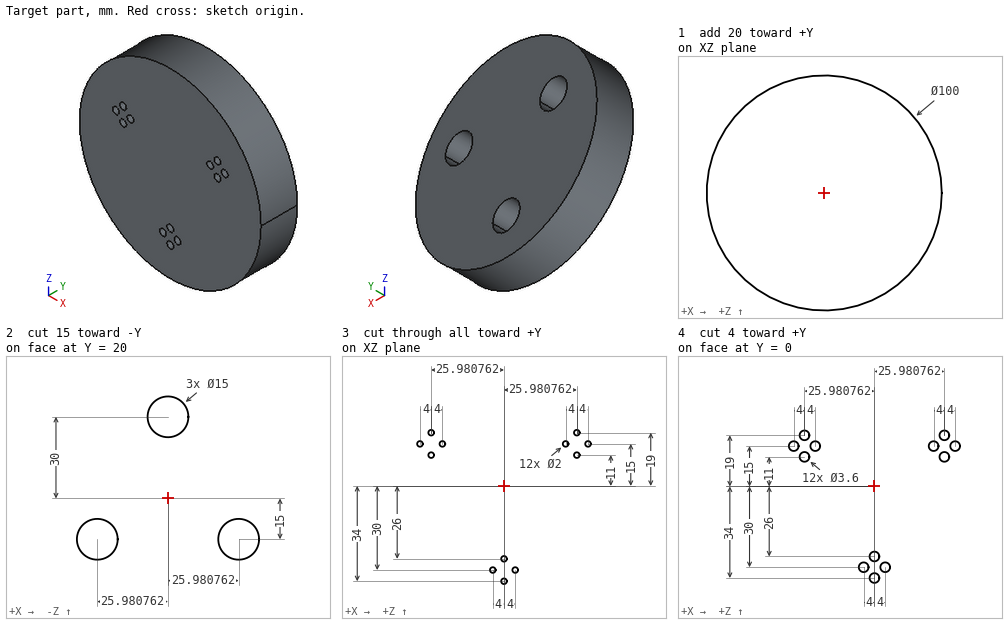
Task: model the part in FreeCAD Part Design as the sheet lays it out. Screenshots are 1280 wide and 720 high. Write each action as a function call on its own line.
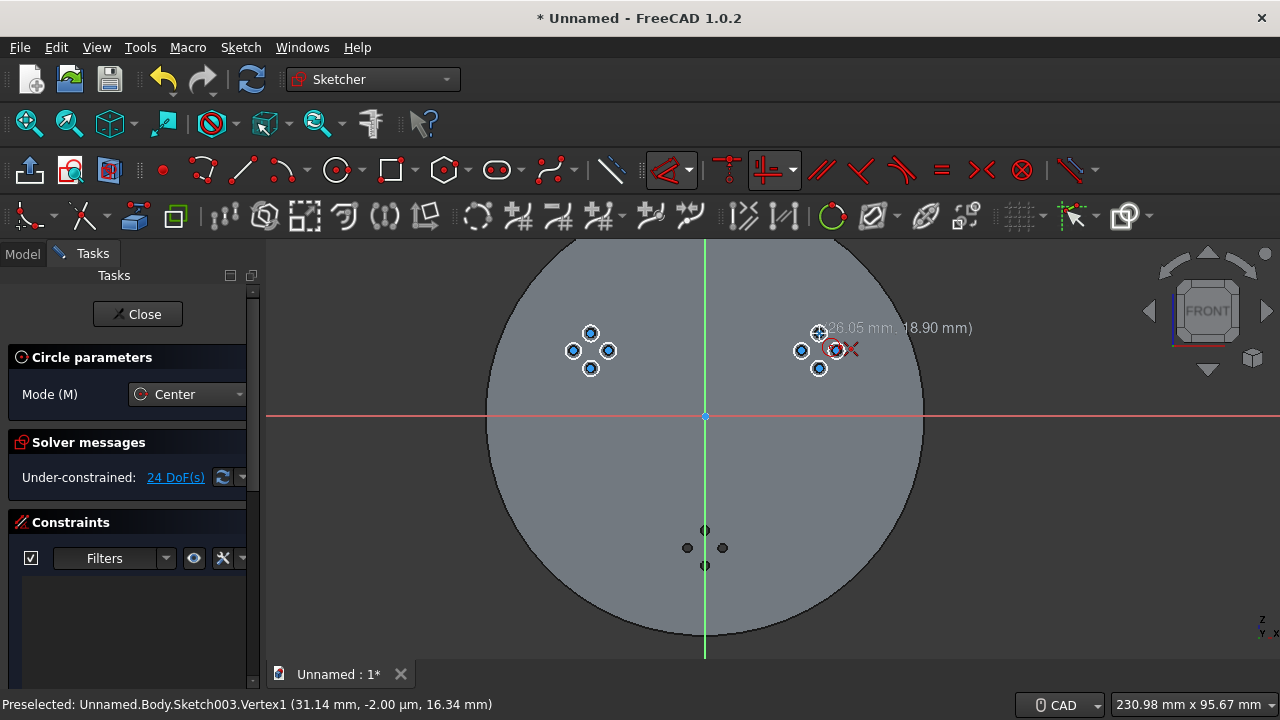
scroll(705, 531, up, 6)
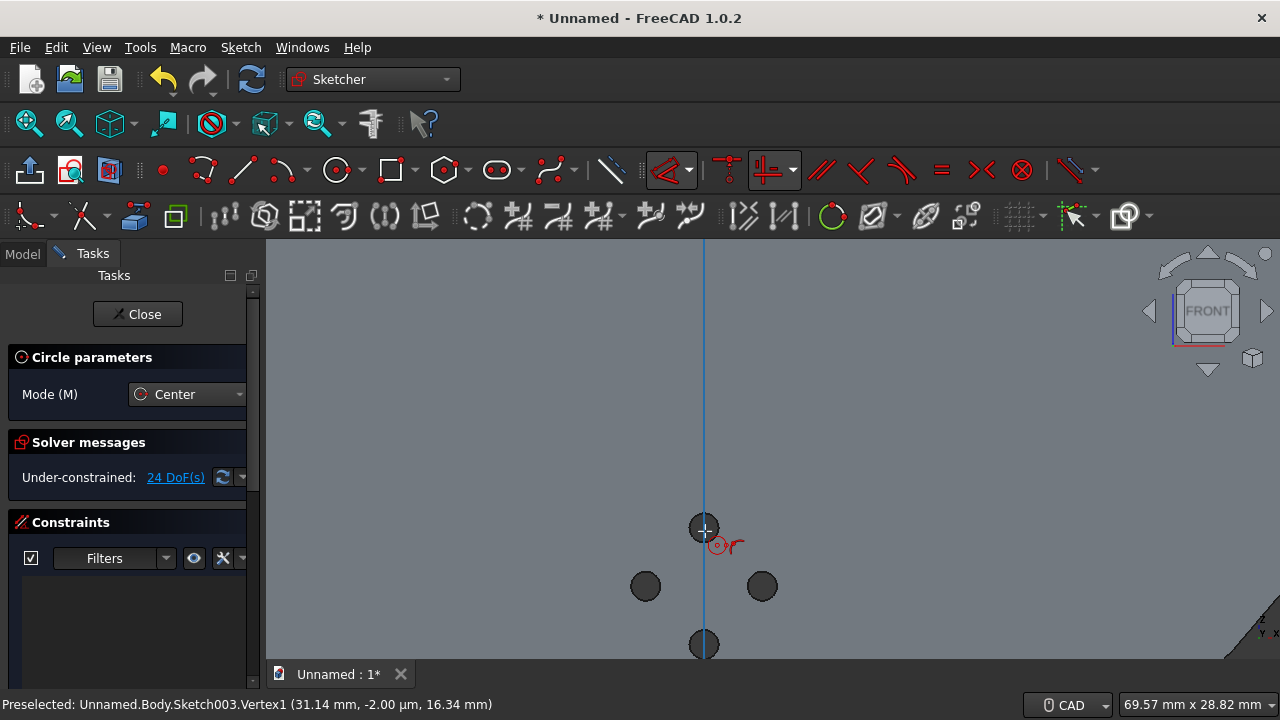
click(704, 528)
click(723, 509)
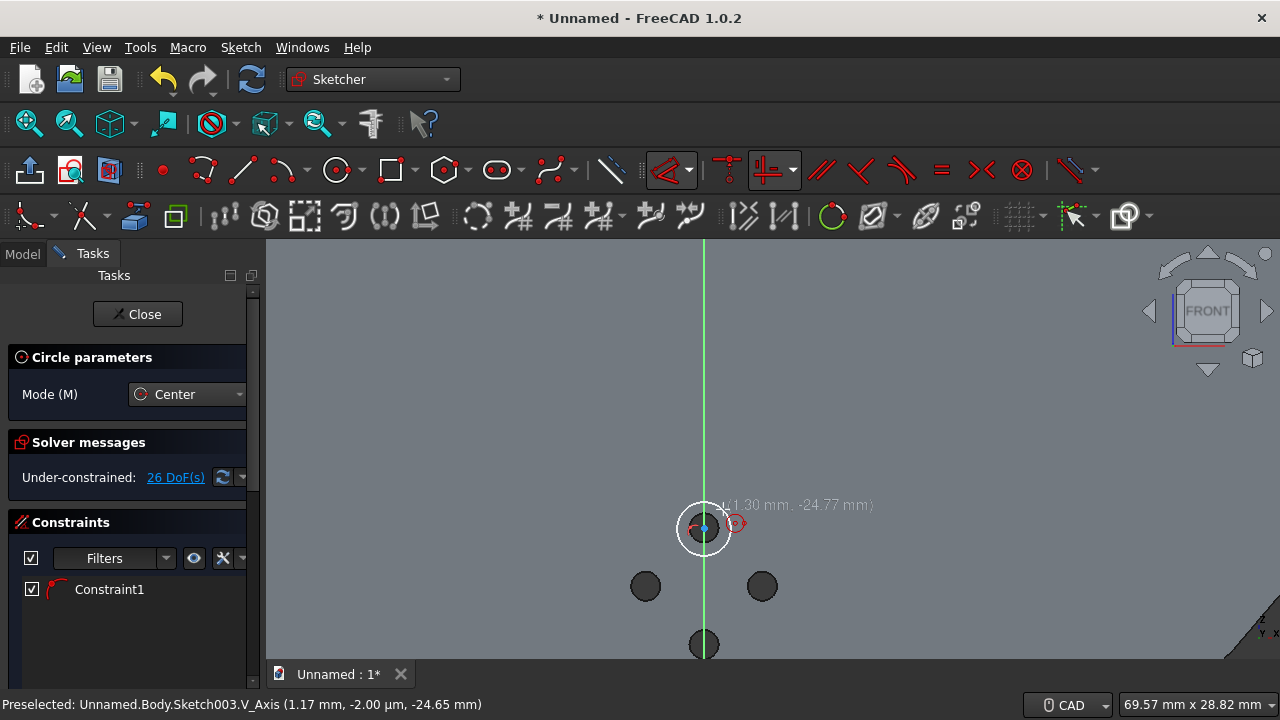
click(646, 586)
click(664, 568)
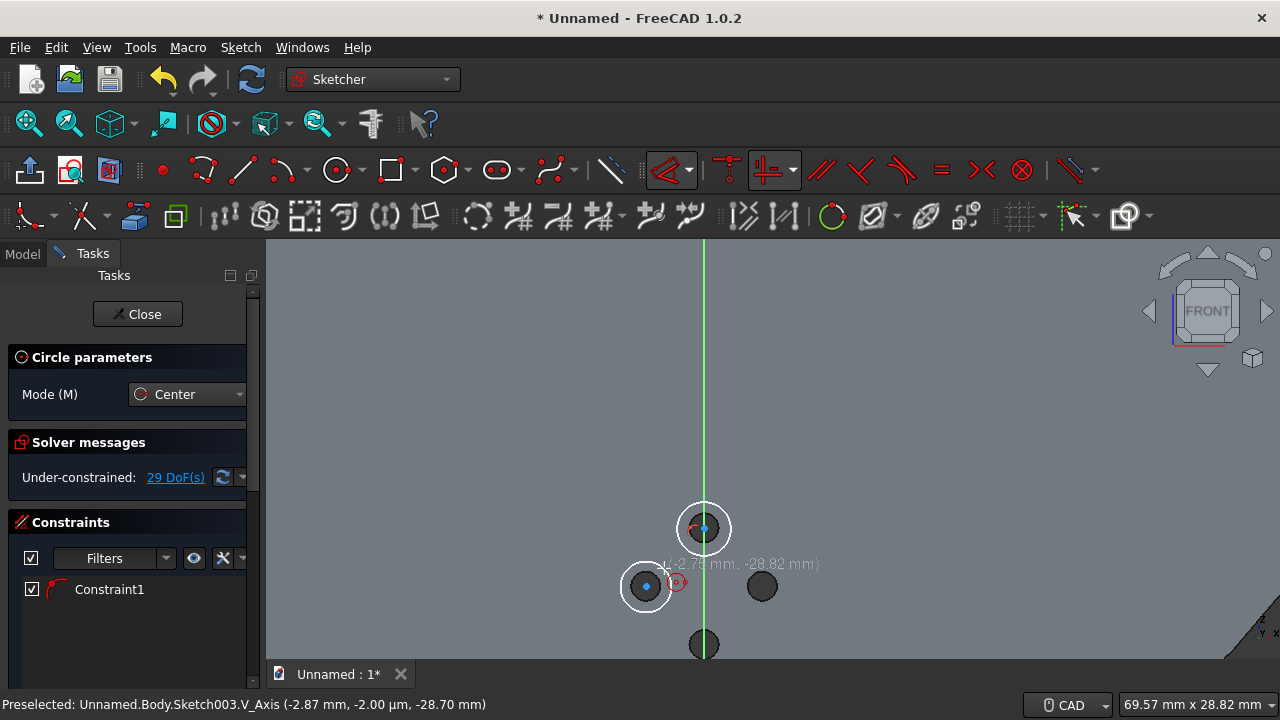
scroll(705, 531, down, 6)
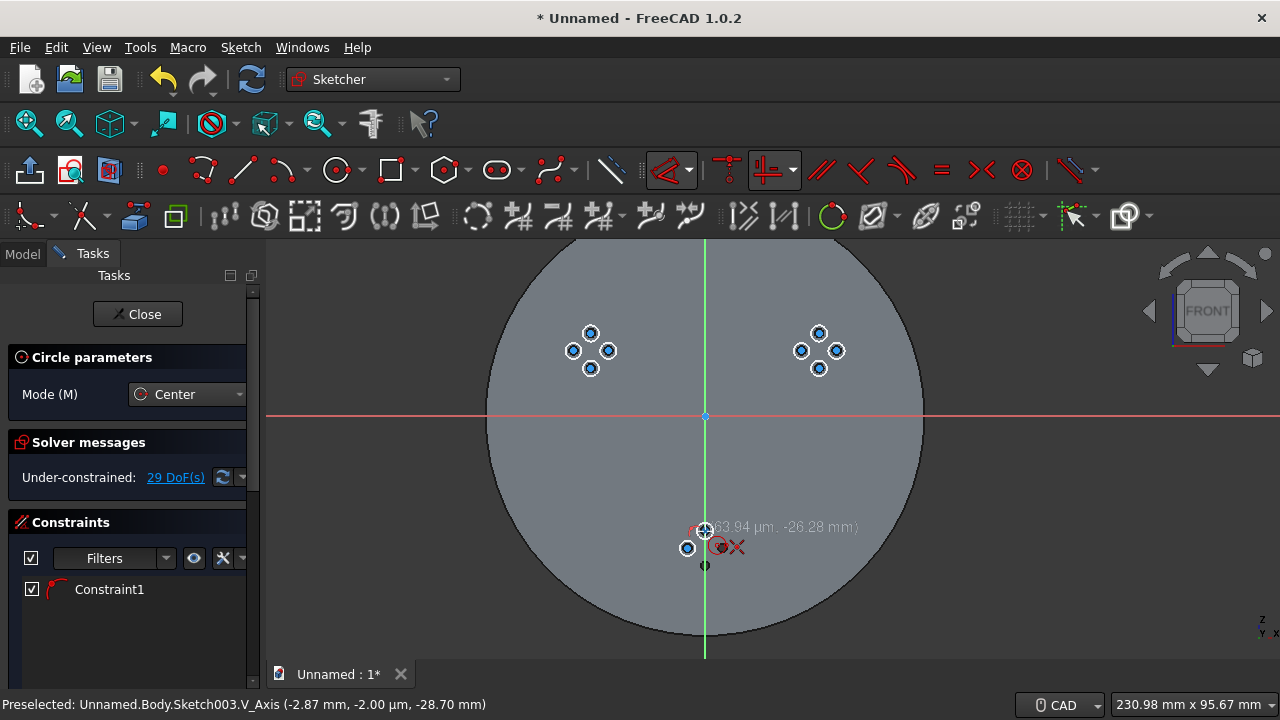
scroll(705, 566, up, 6)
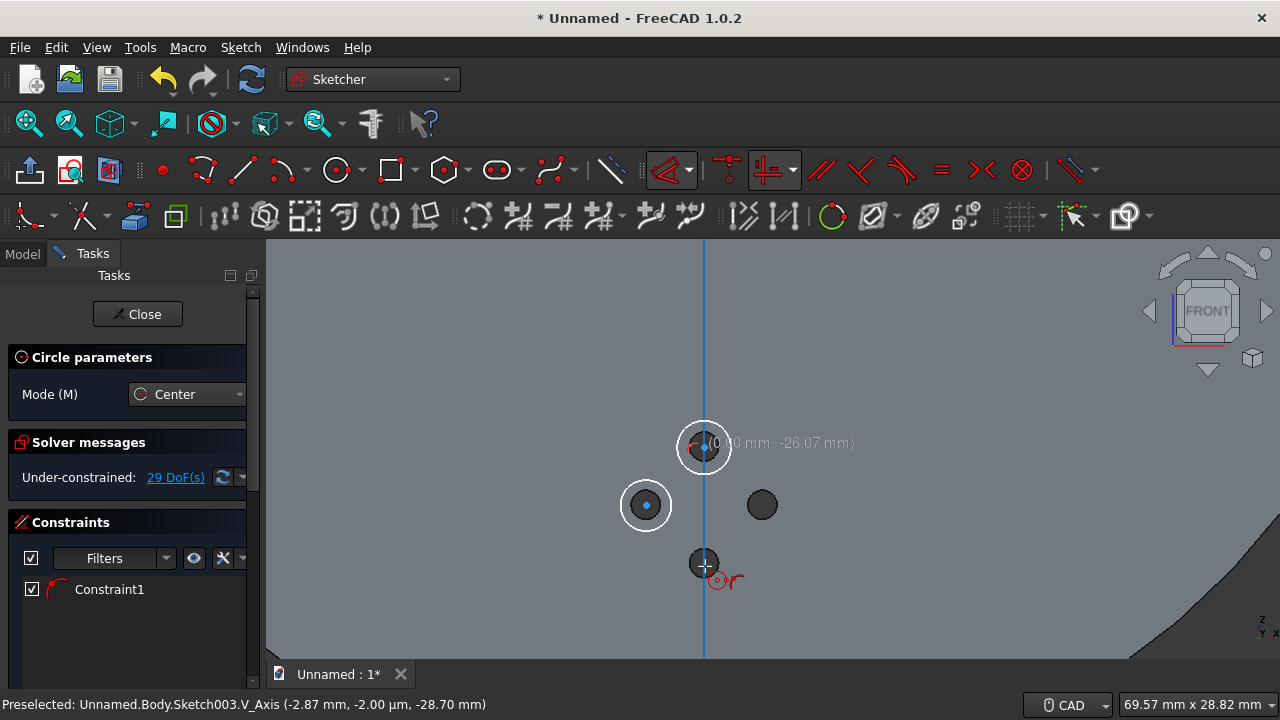
click(704, 563)
click(723, 545)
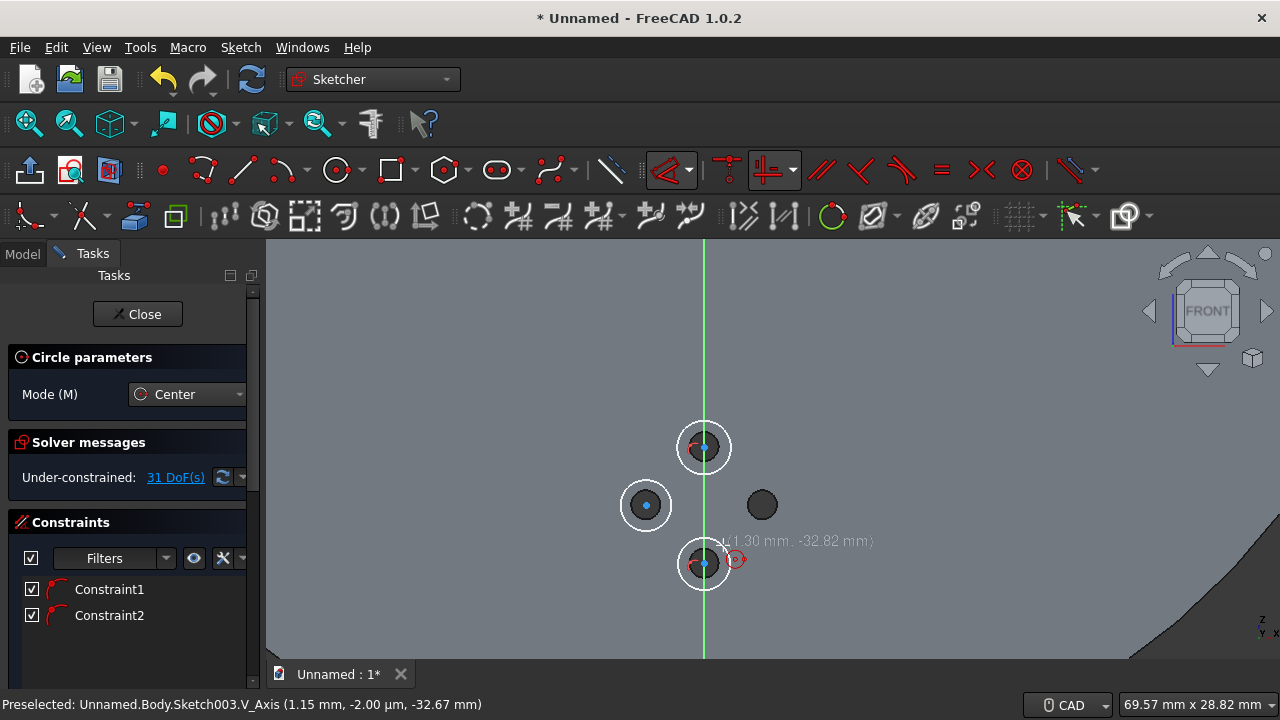
click(762, 505)
click(781, 486)
key(Escape)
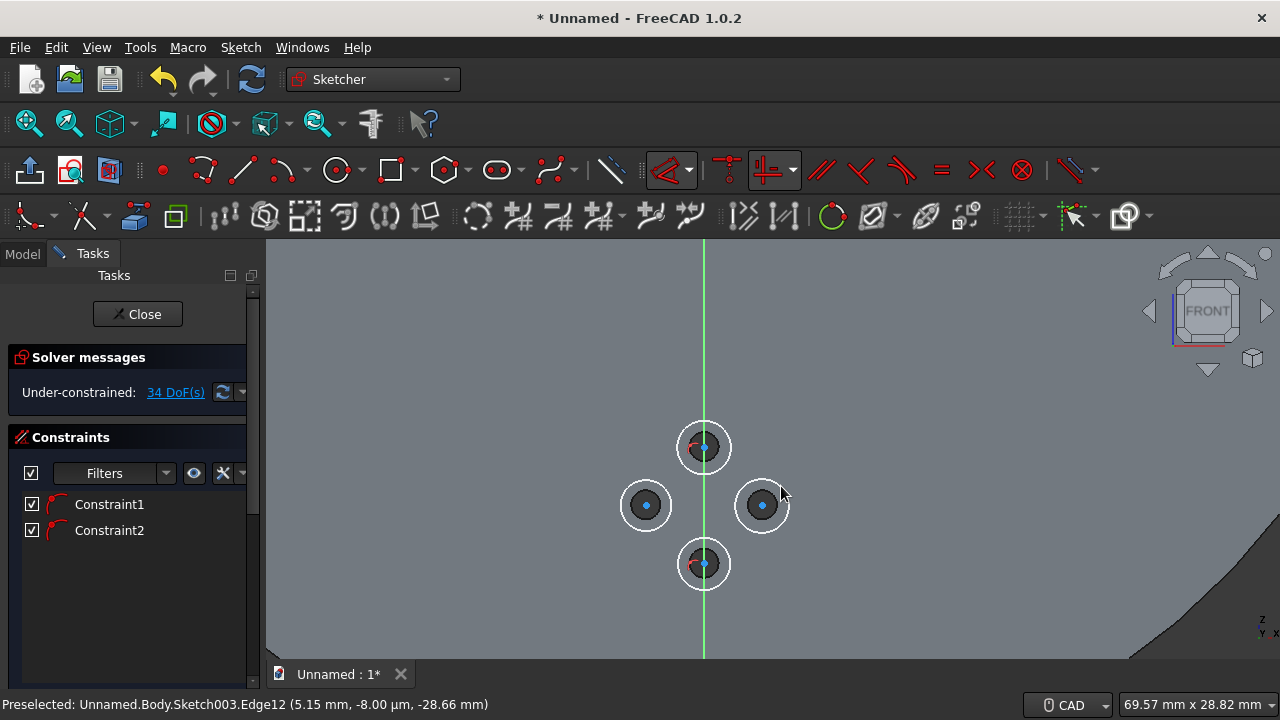
scroll(705, 566, down, 6)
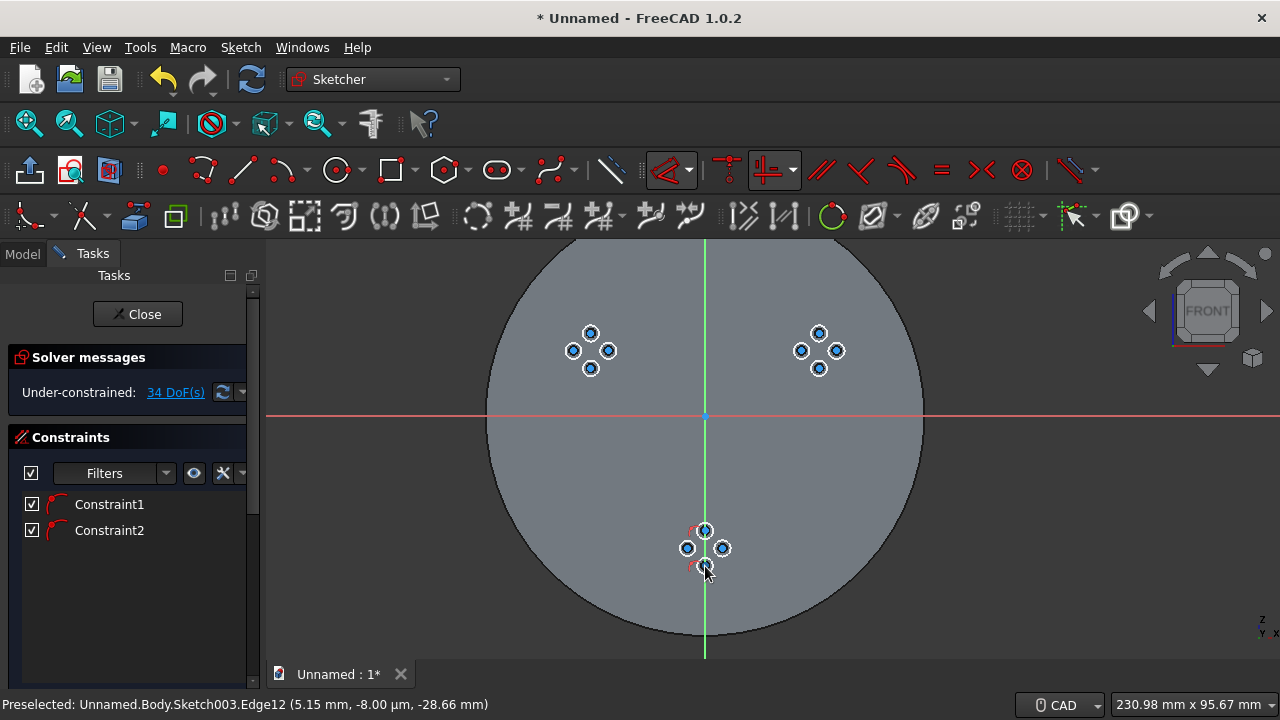
scroll(597, 328, up, 3)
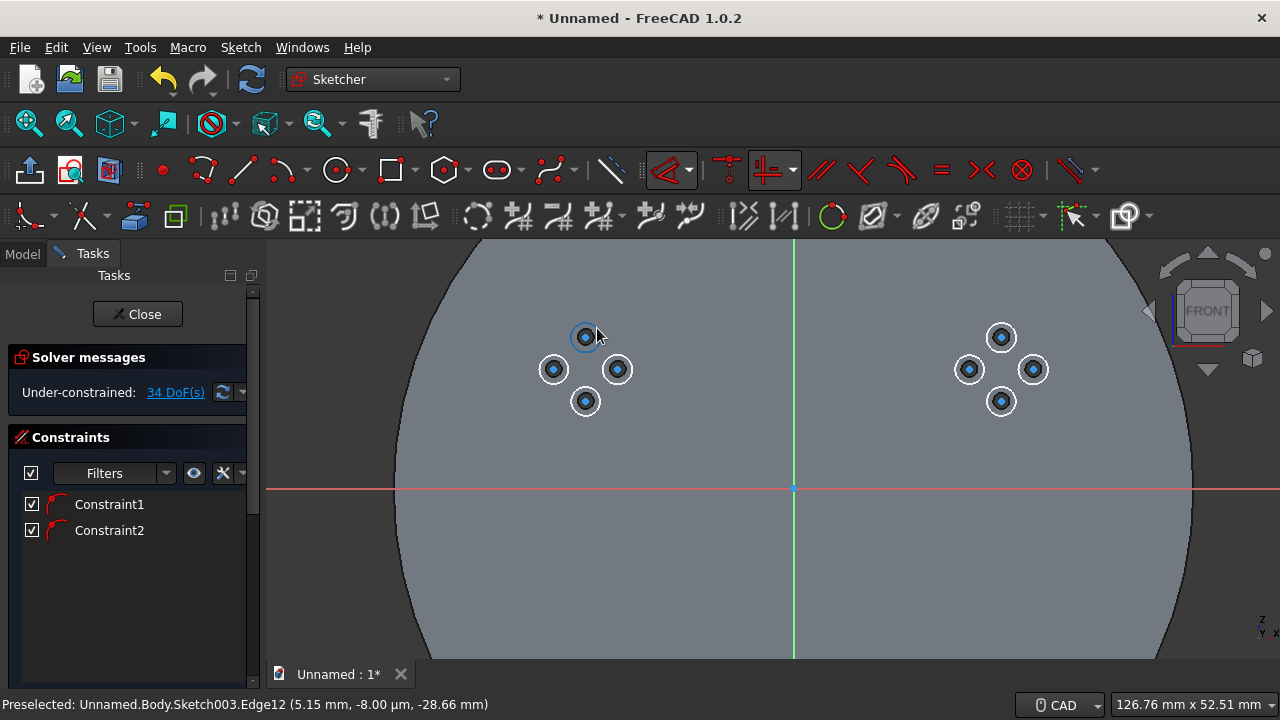
click(596, 327)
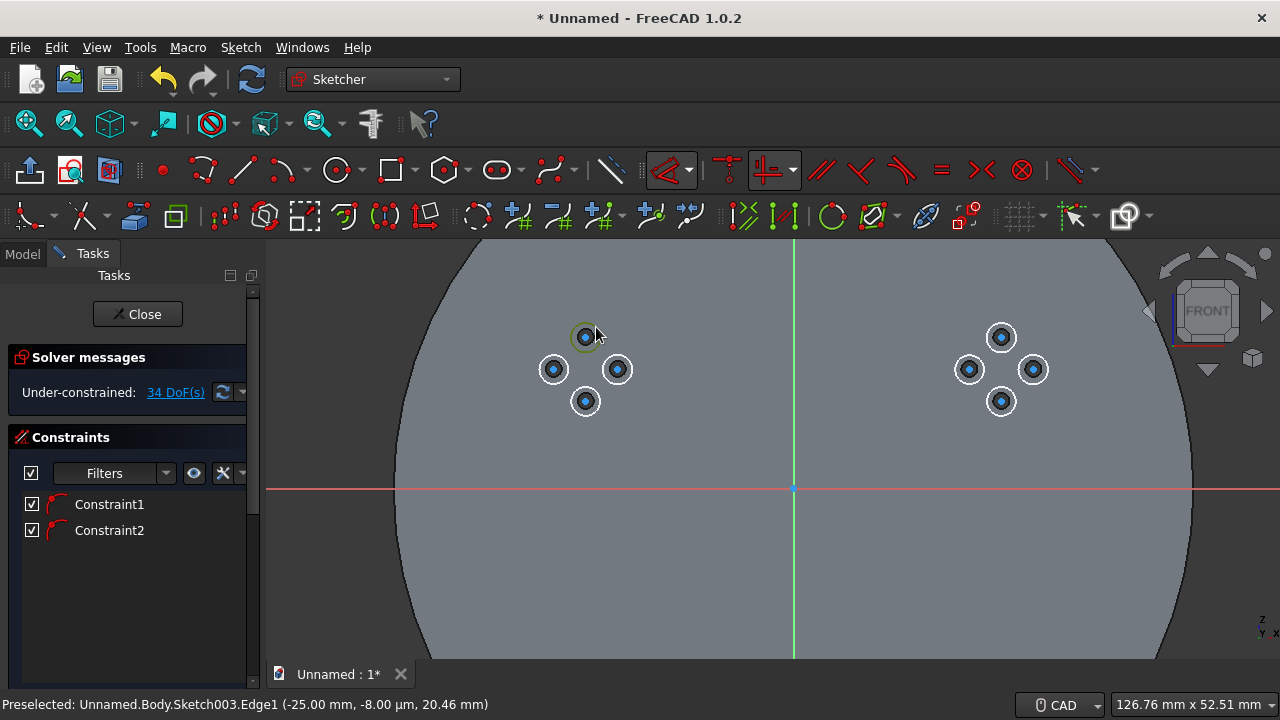
click(564, 359)